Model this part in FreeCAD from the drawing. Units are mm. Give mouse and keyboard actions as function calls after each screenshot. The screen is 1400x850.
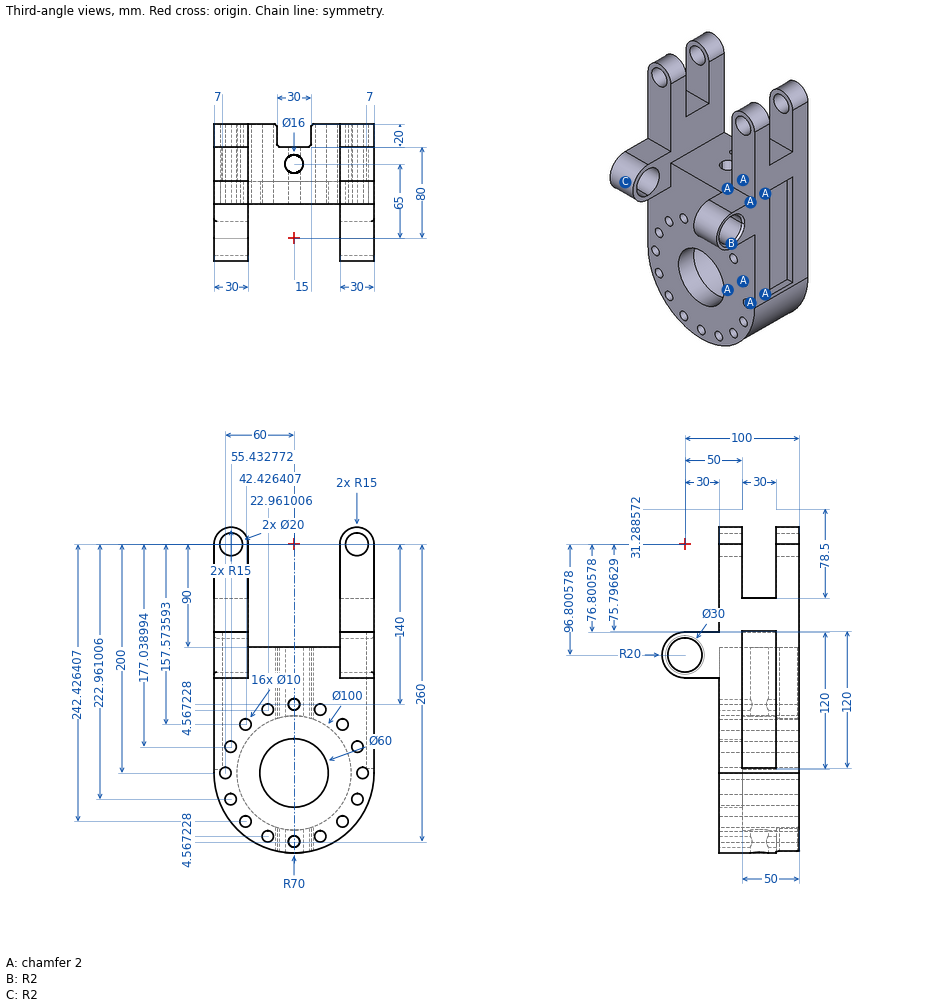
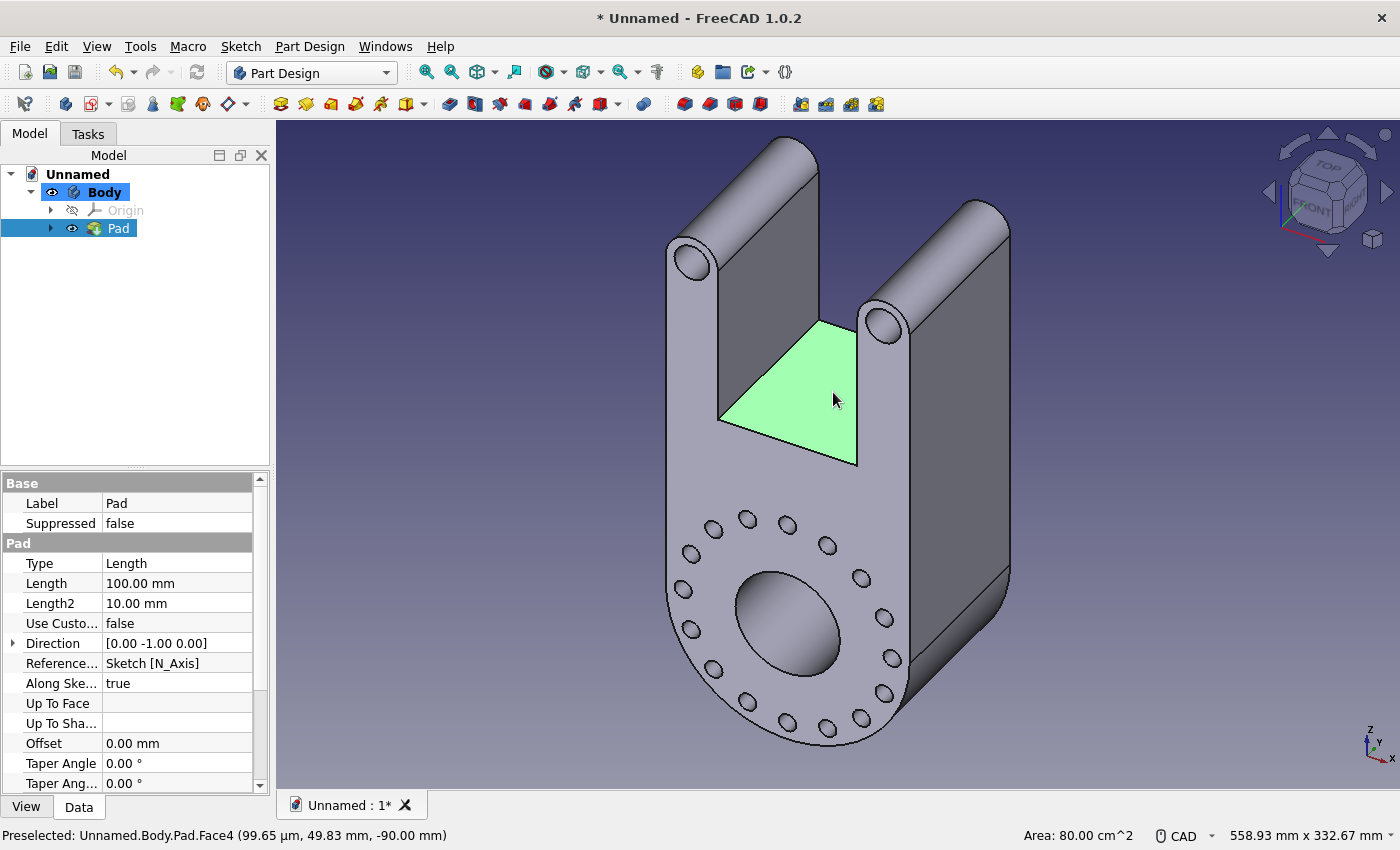
click(90, 104)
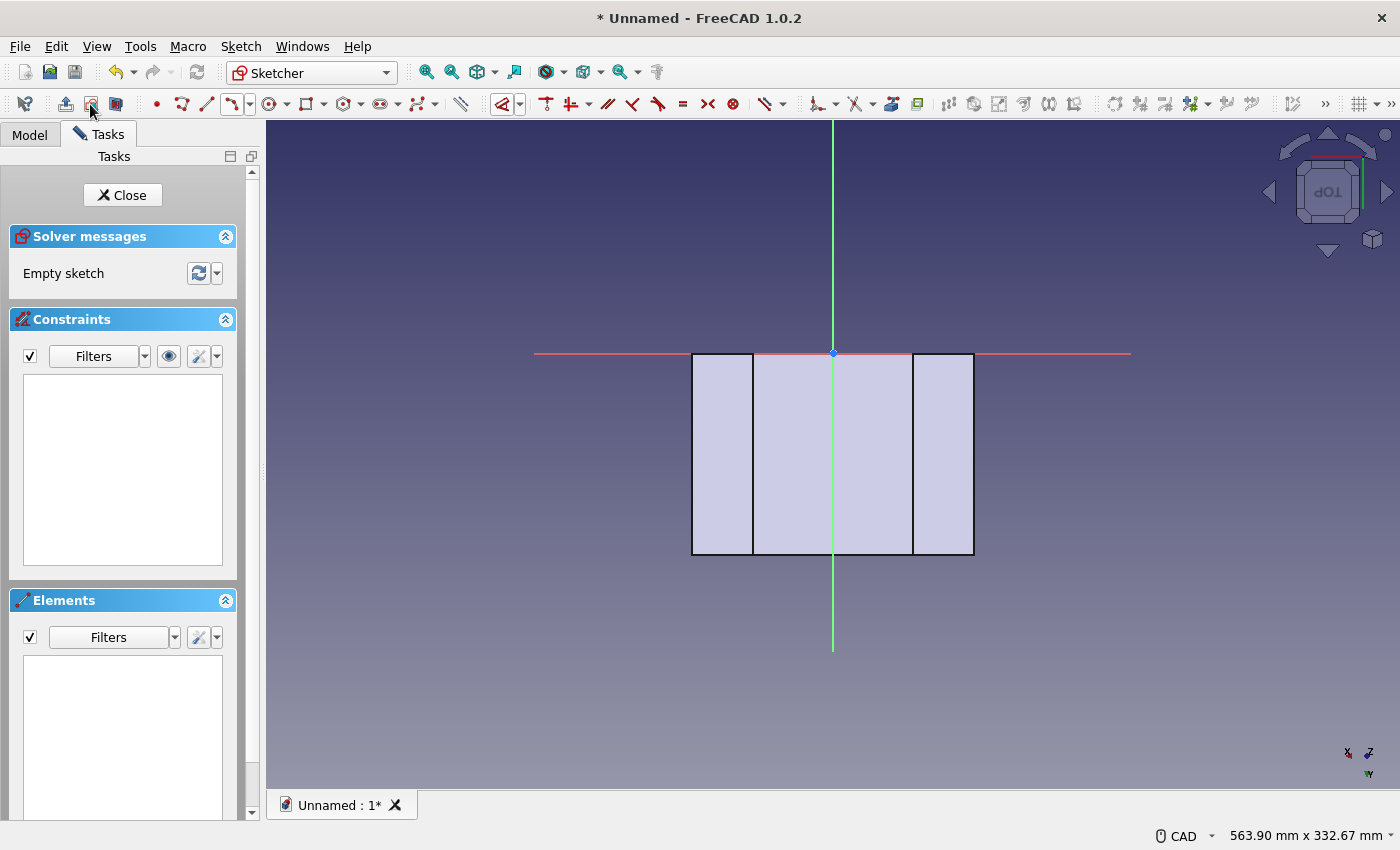
click(116, 104)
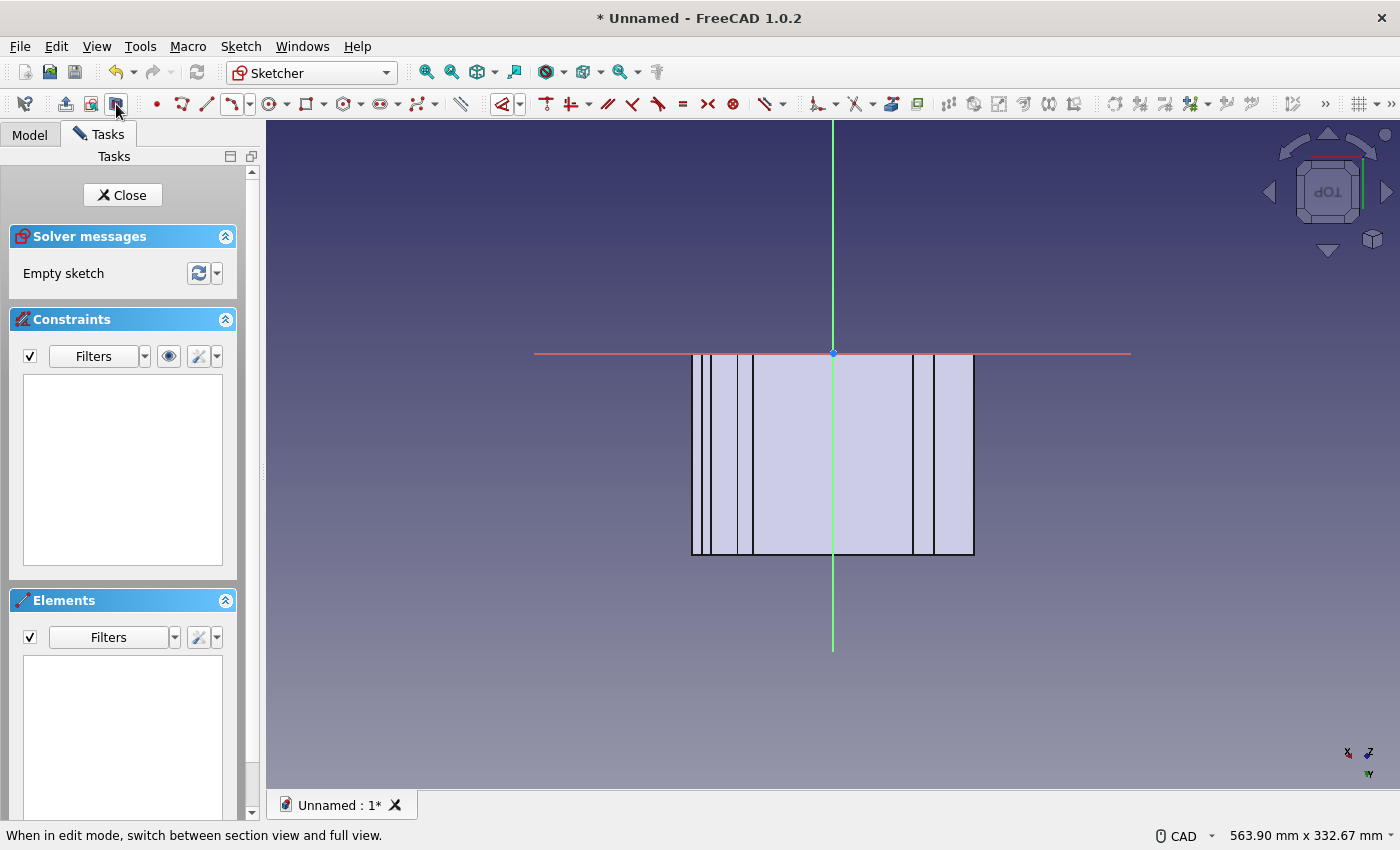
scroll(840, 543, up, 12)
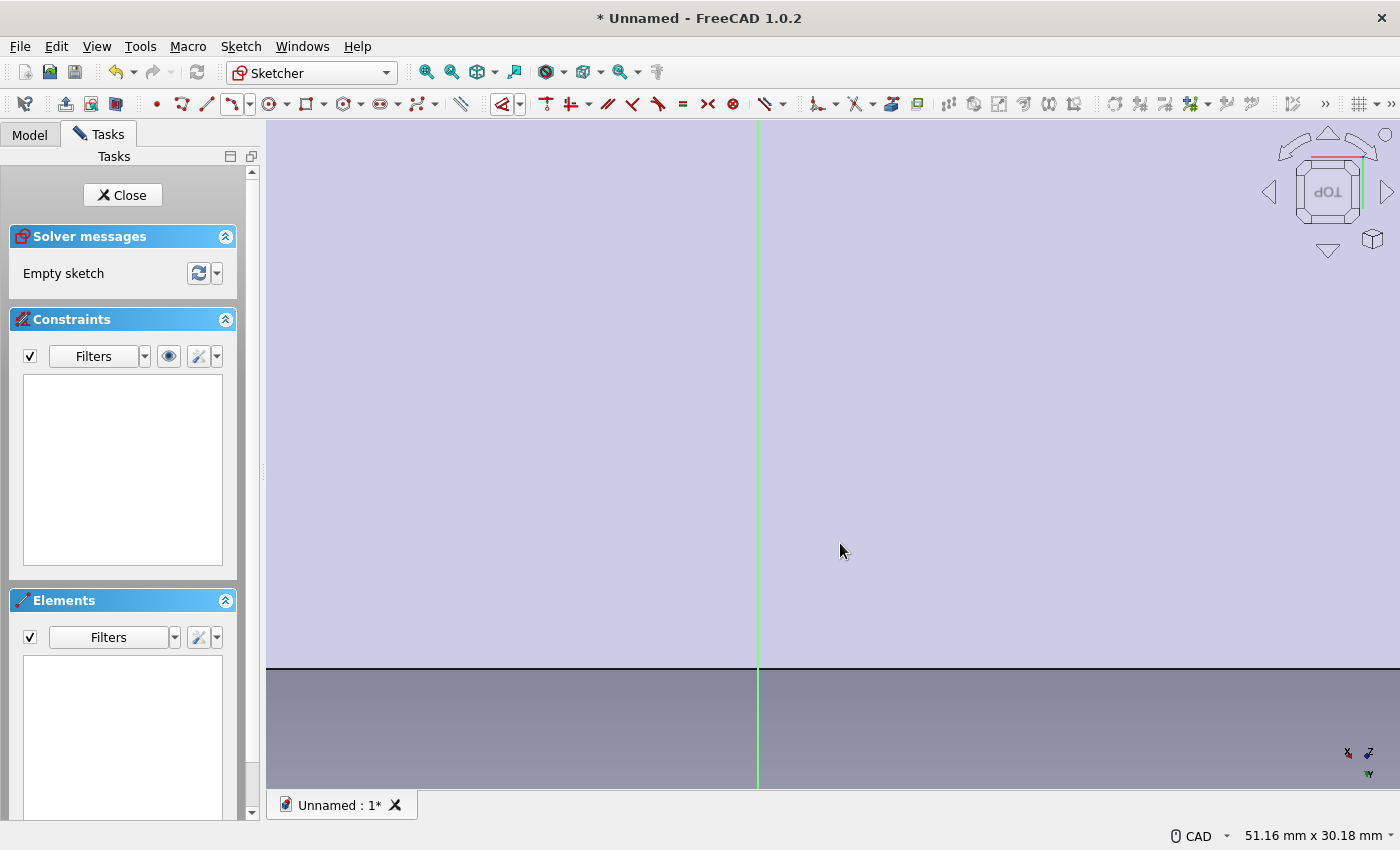
key(g)
key(r)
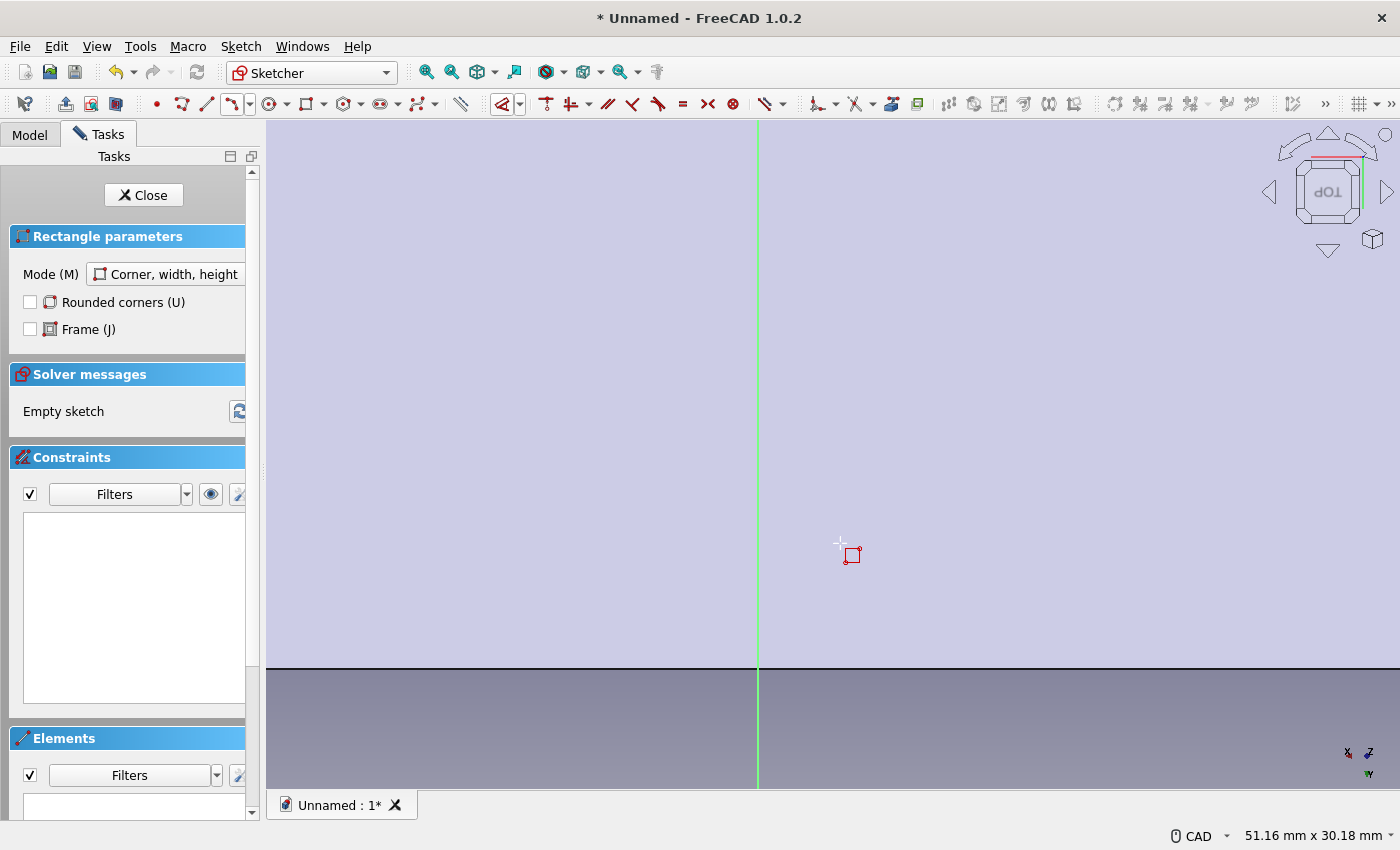
click(425, 226)
click(1090, 669)
key(Escape)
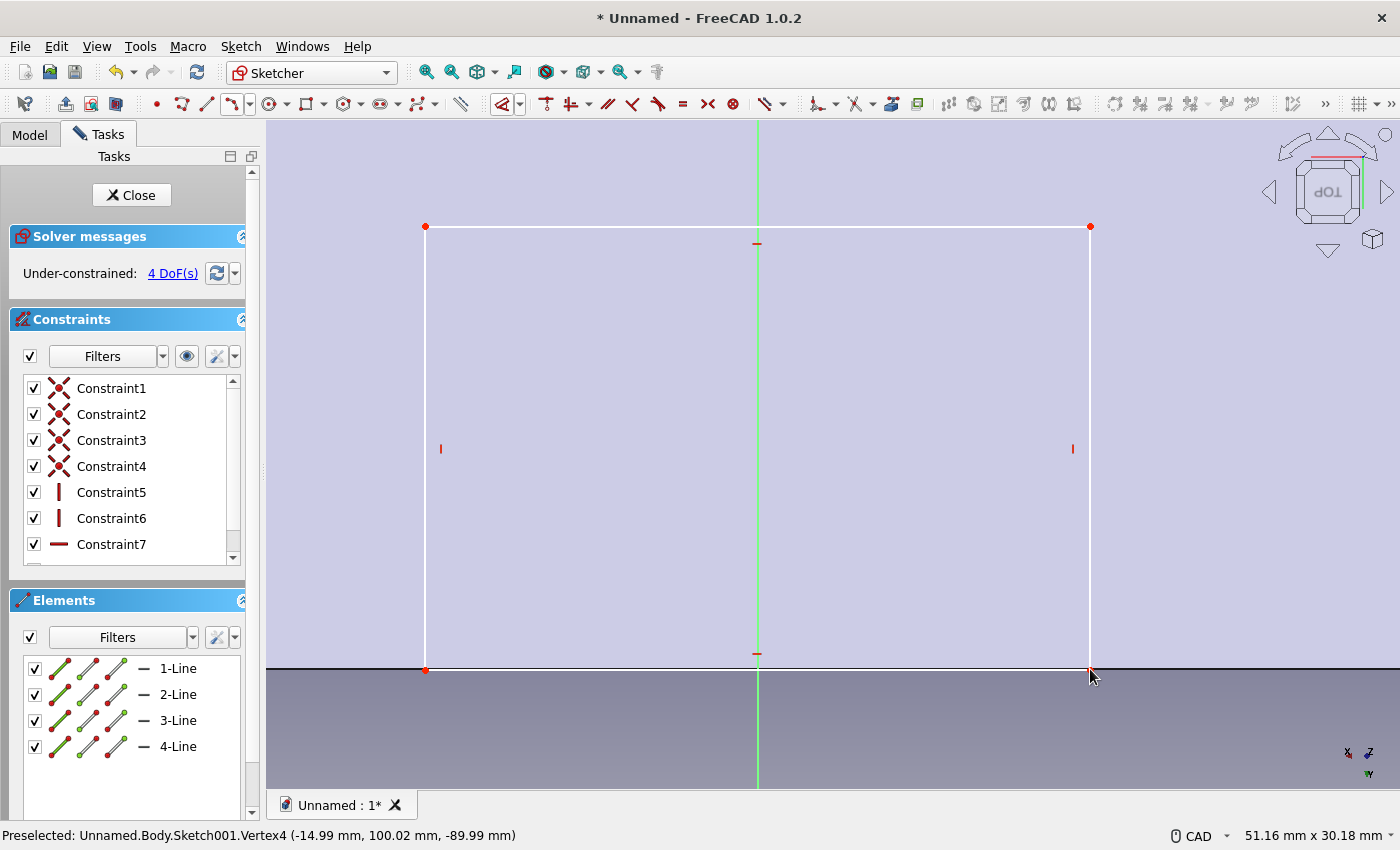
click(502, 104)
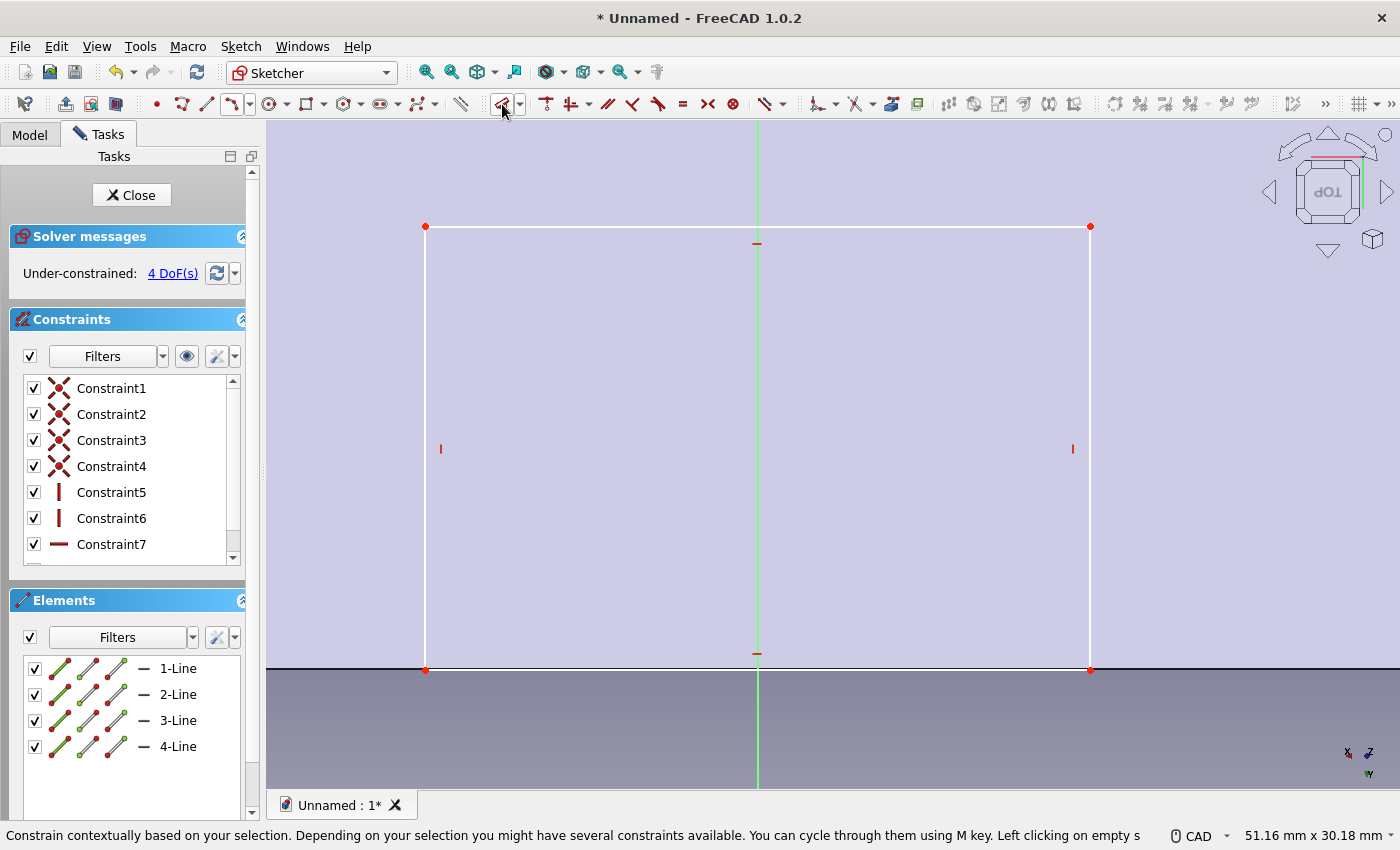
click(425, 360)
click(391, 449)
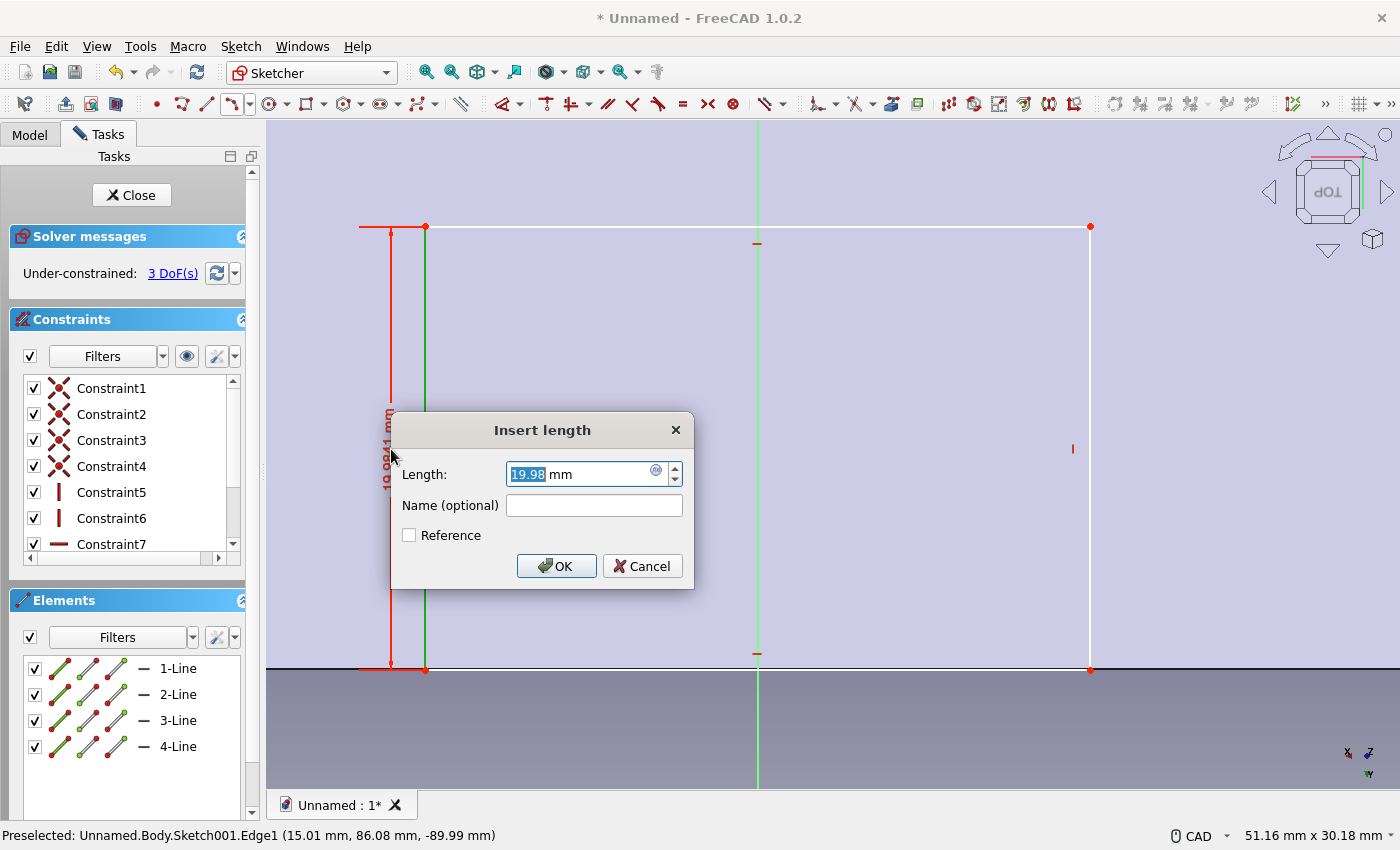
text(20)
key(Return)